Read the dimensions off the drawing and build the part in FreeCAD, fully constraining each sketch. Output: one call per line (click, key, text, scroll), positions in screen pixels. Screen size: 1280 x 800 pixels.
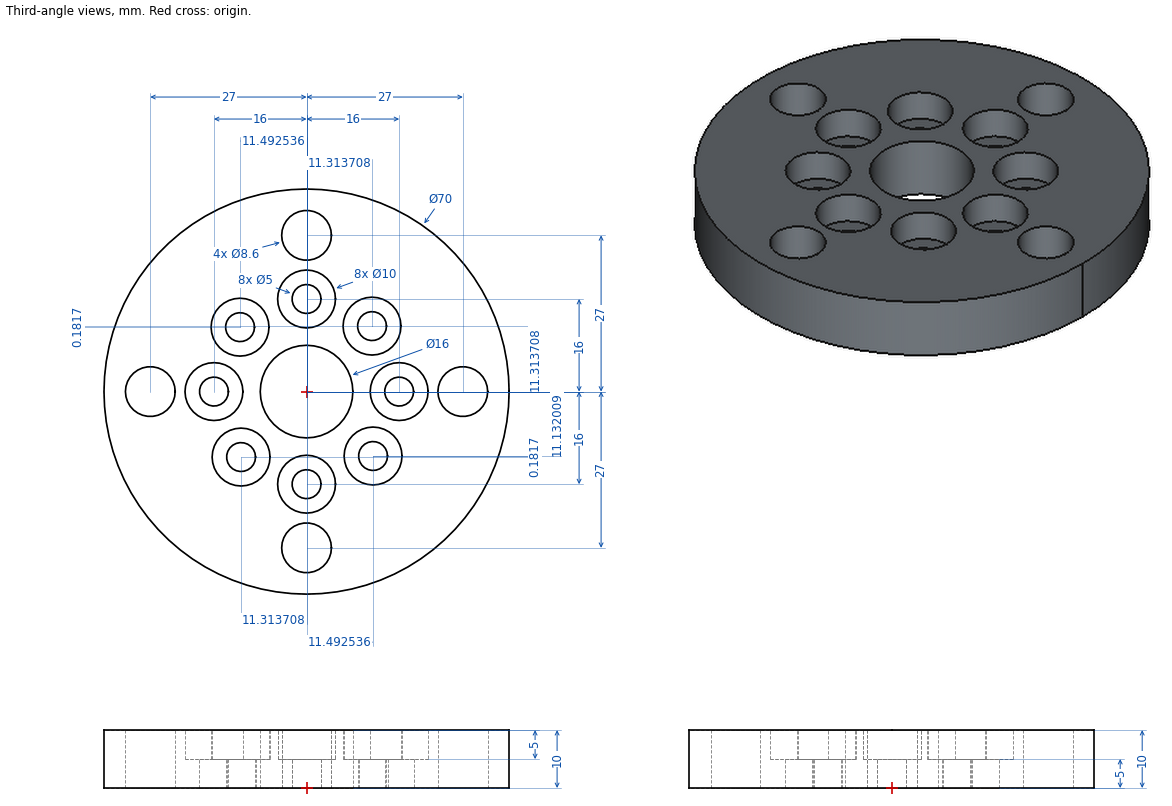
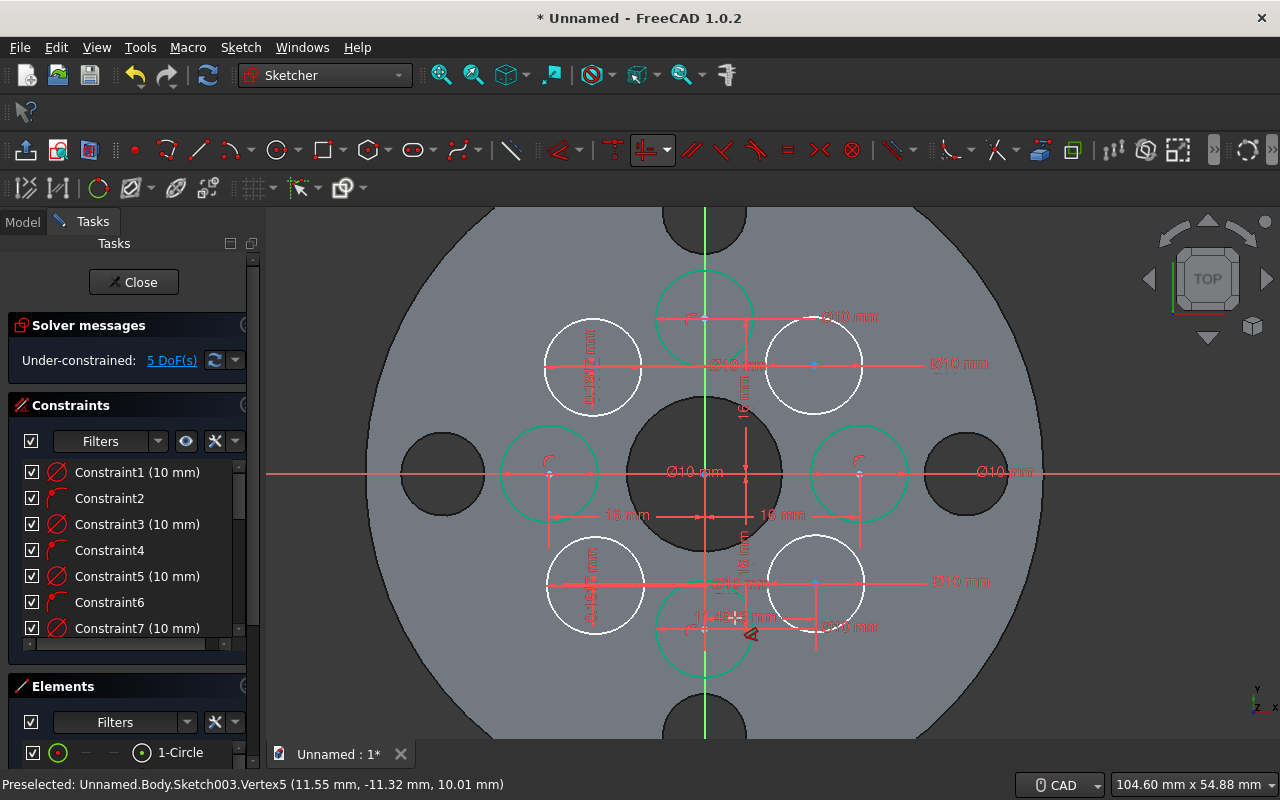
click(816, 584)
click(850, 491)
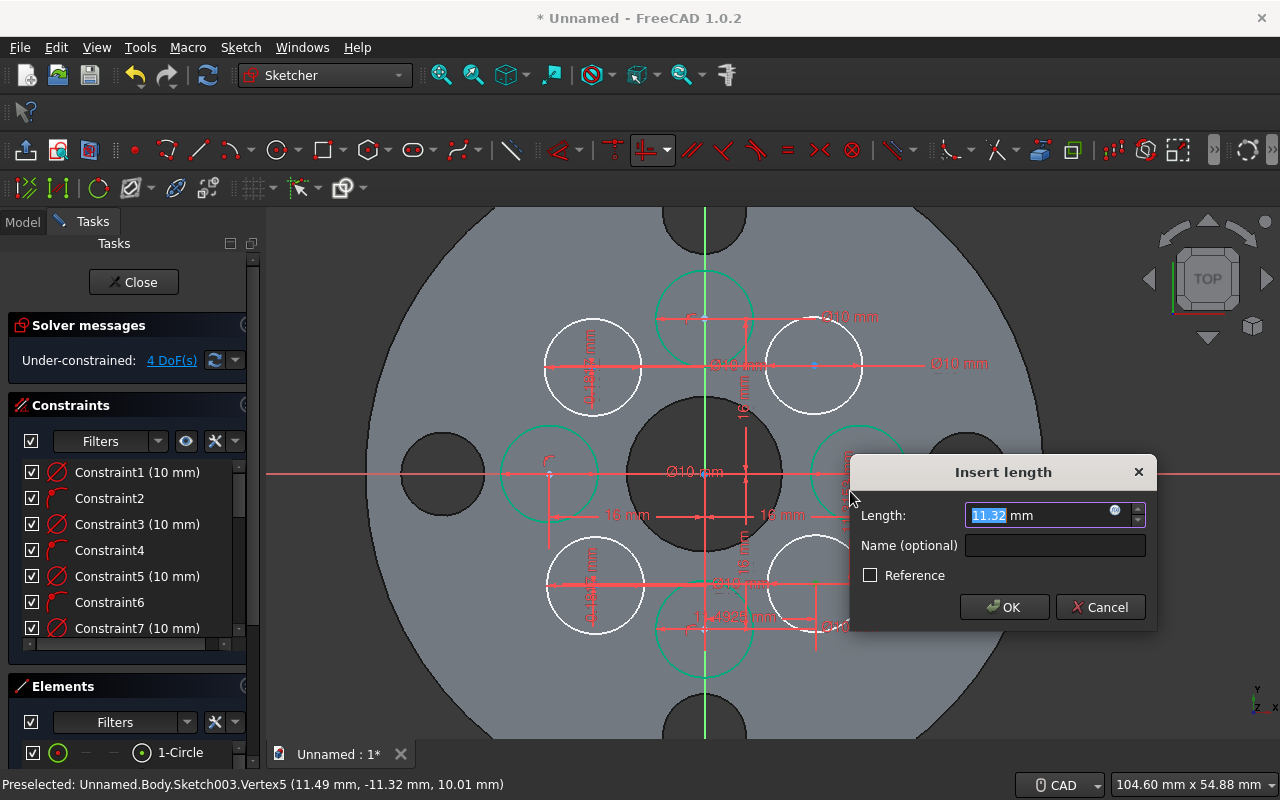
text(11.132009)
key(Return)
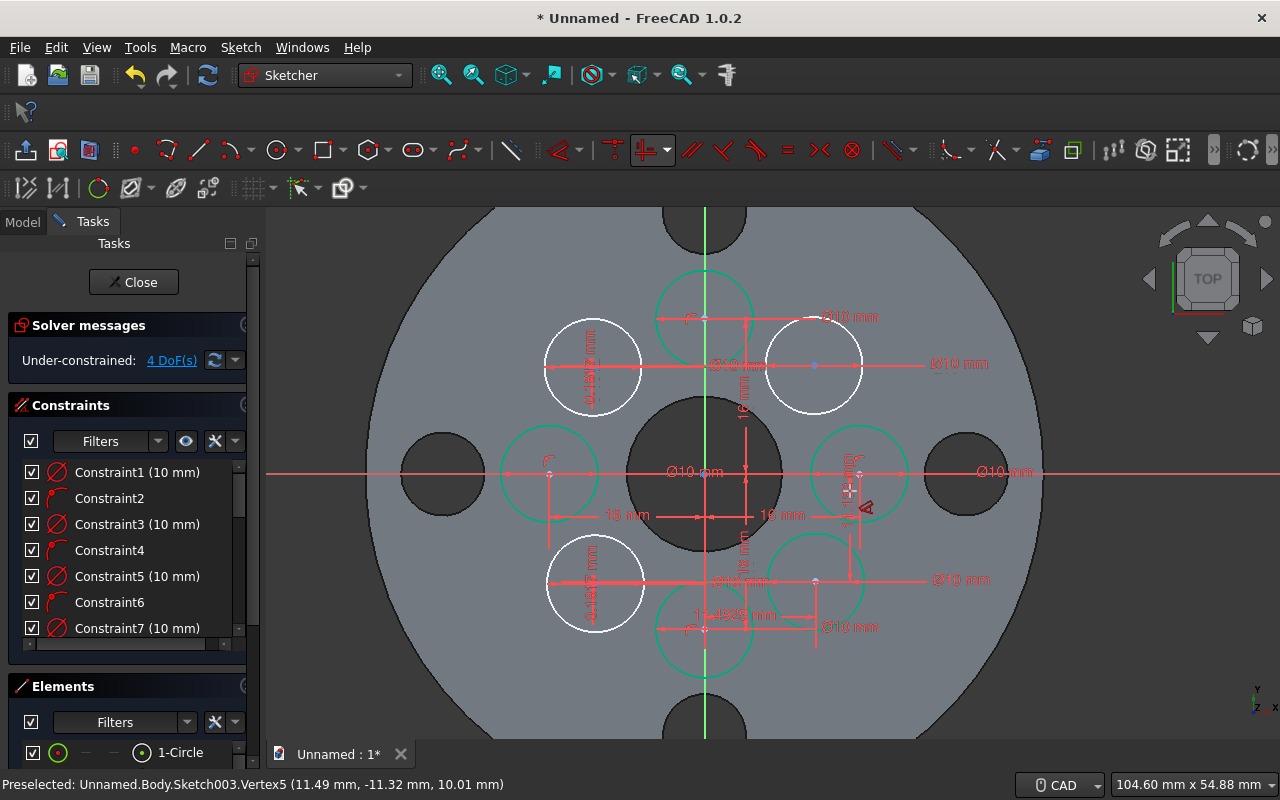
click(814, 366)
click(734, 332)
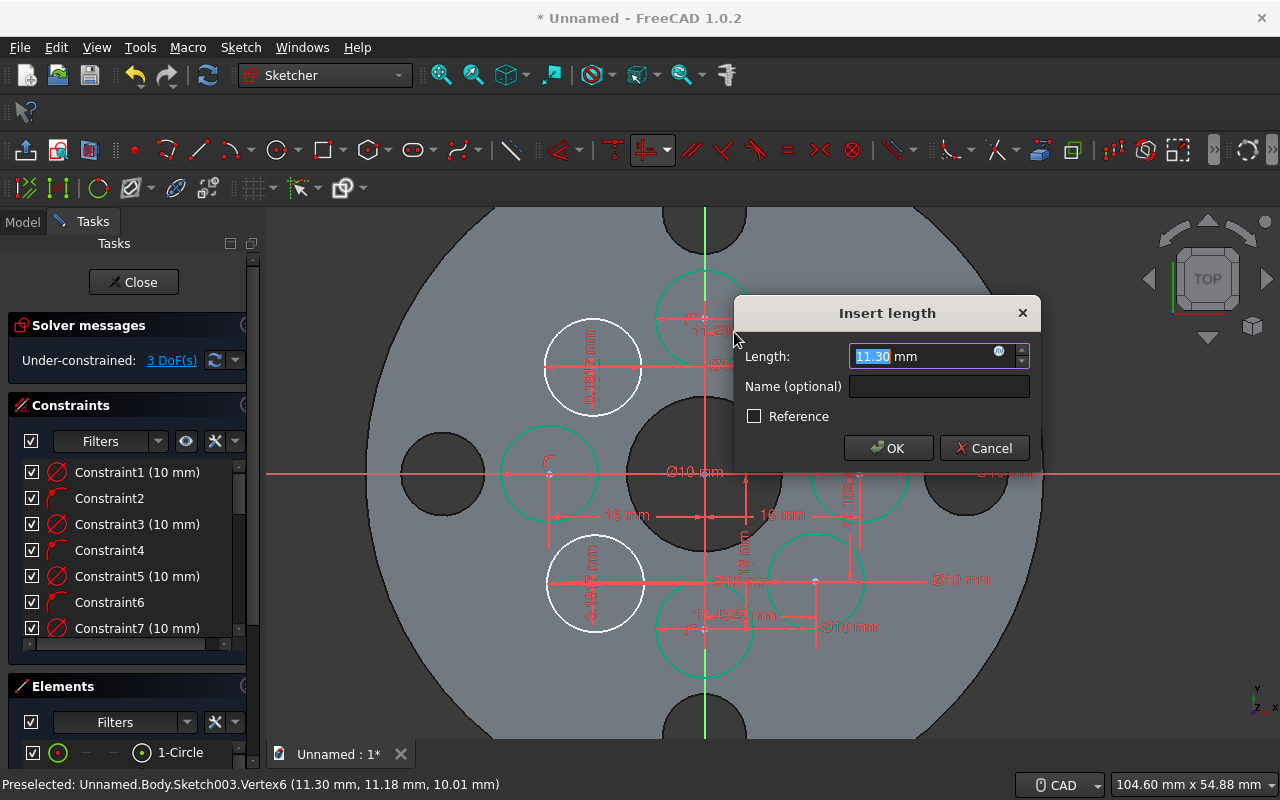
text(11.313708)
key(Return)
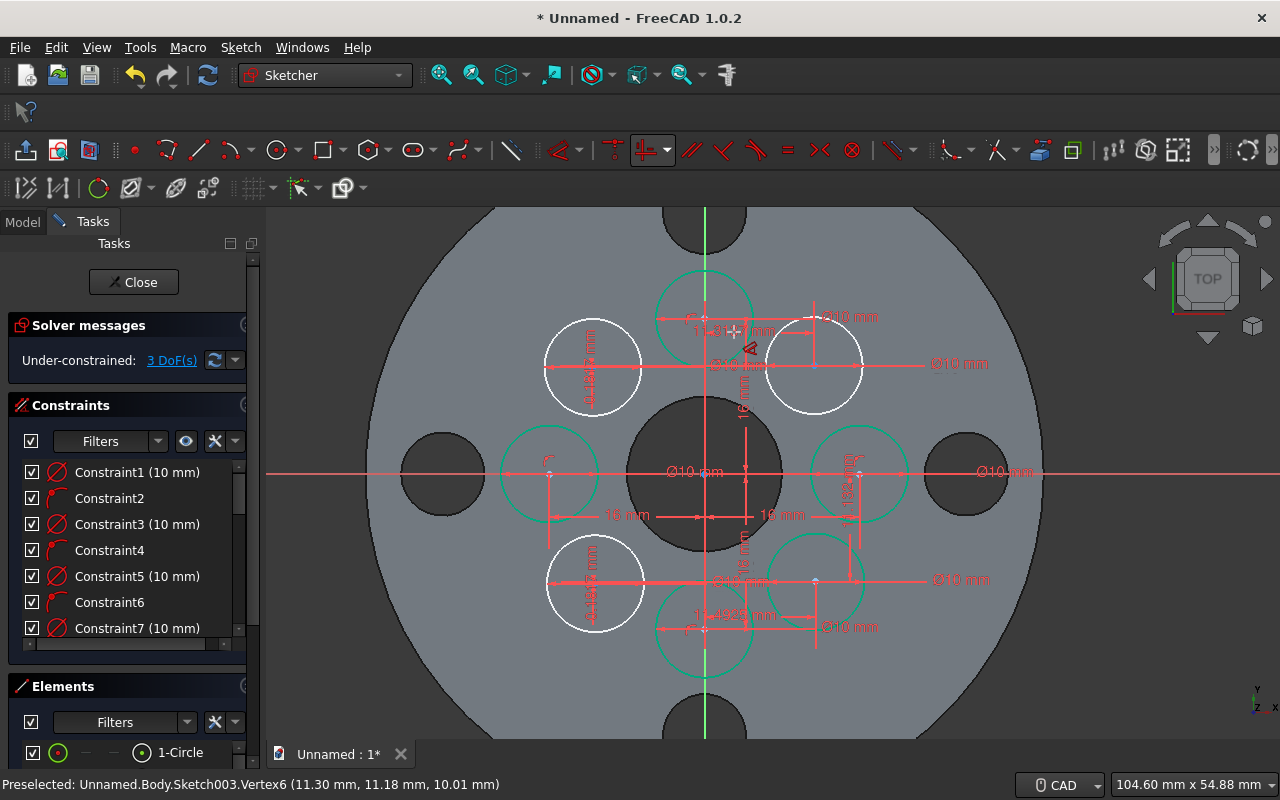
click(814, 366)
click(848, 445)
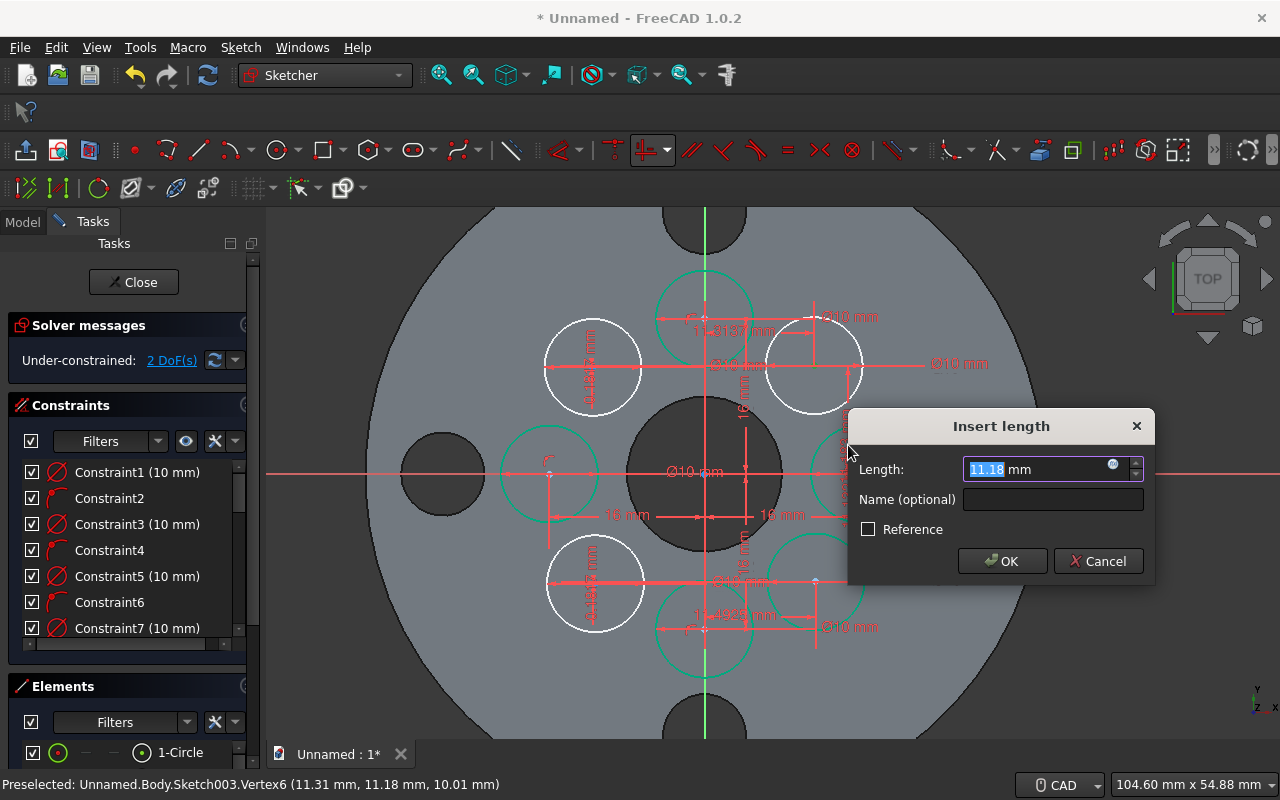
text(11.313708)
key(Return)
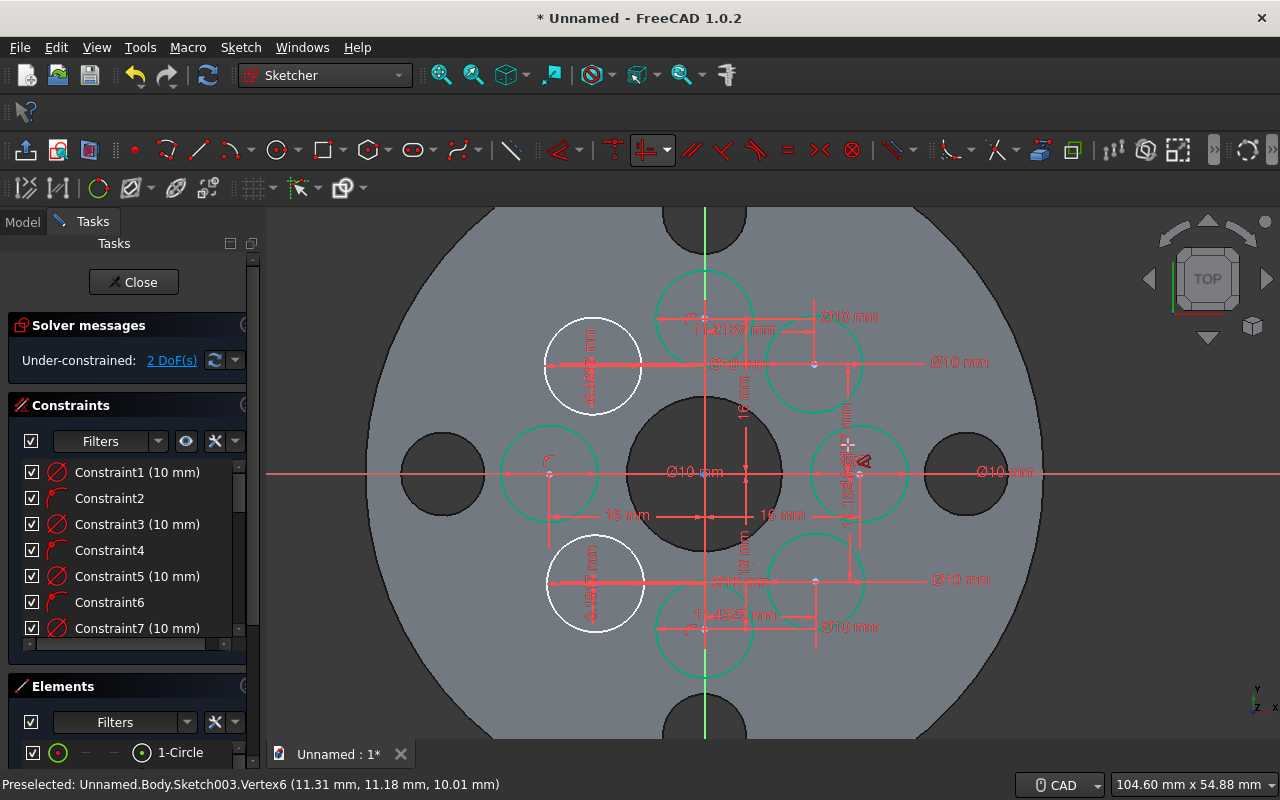
click(593, 366)
click(623, 308)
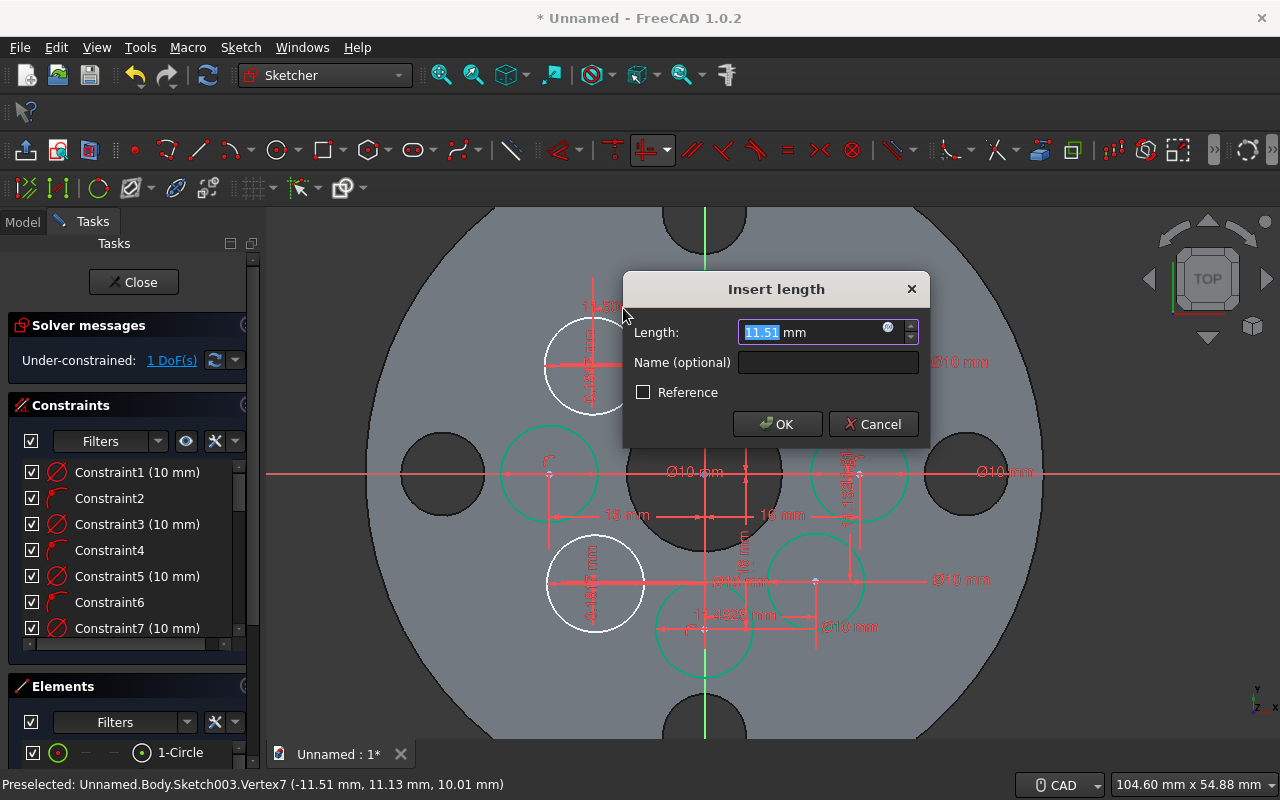
text(11.492536)
key(Return)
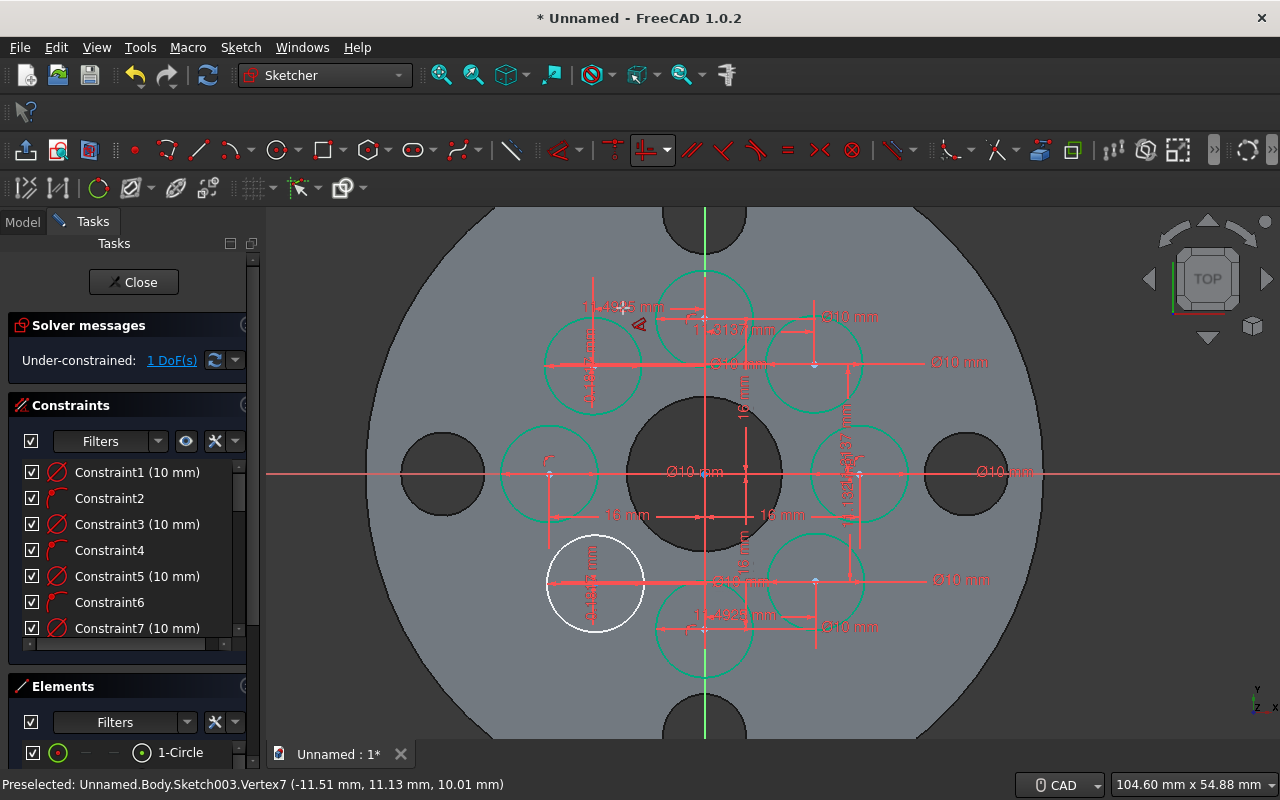
click(595, 584)
click(650, 440)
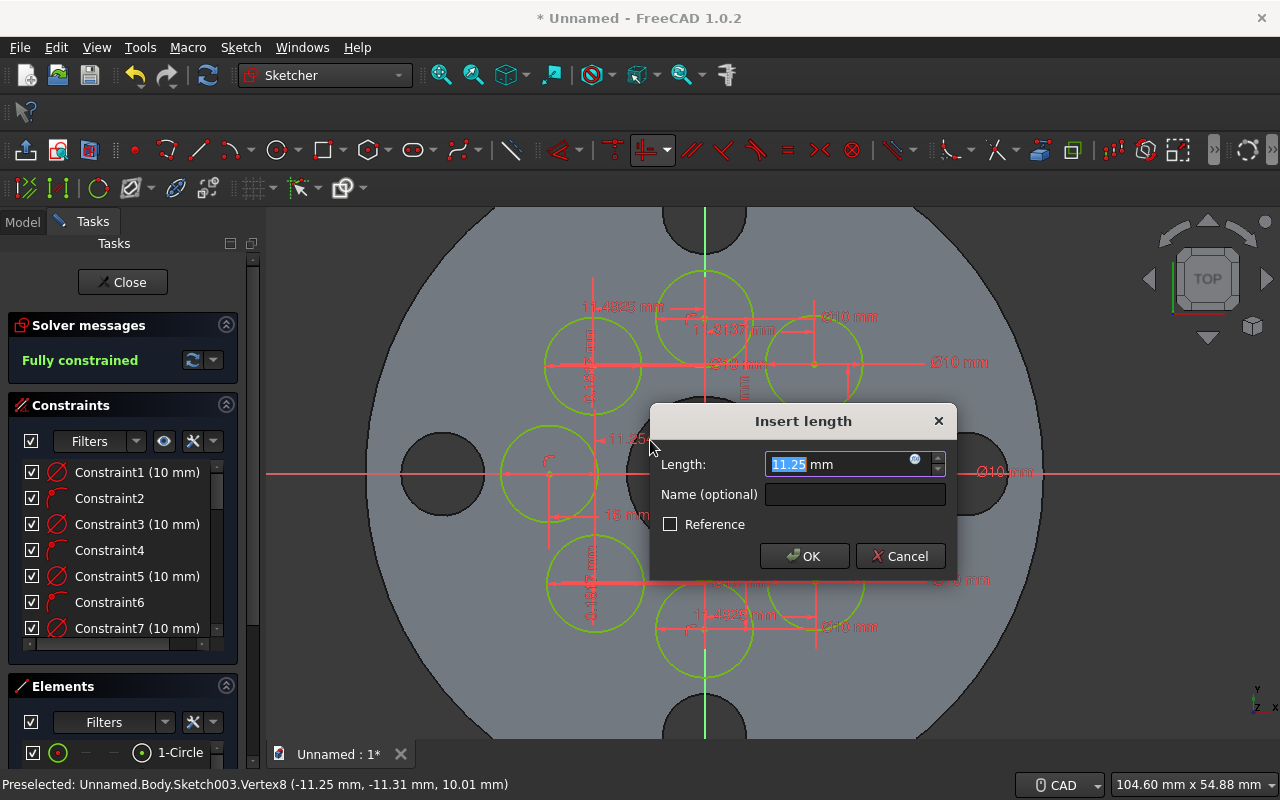
text(11.313708)
key(Return)
key(Escape)